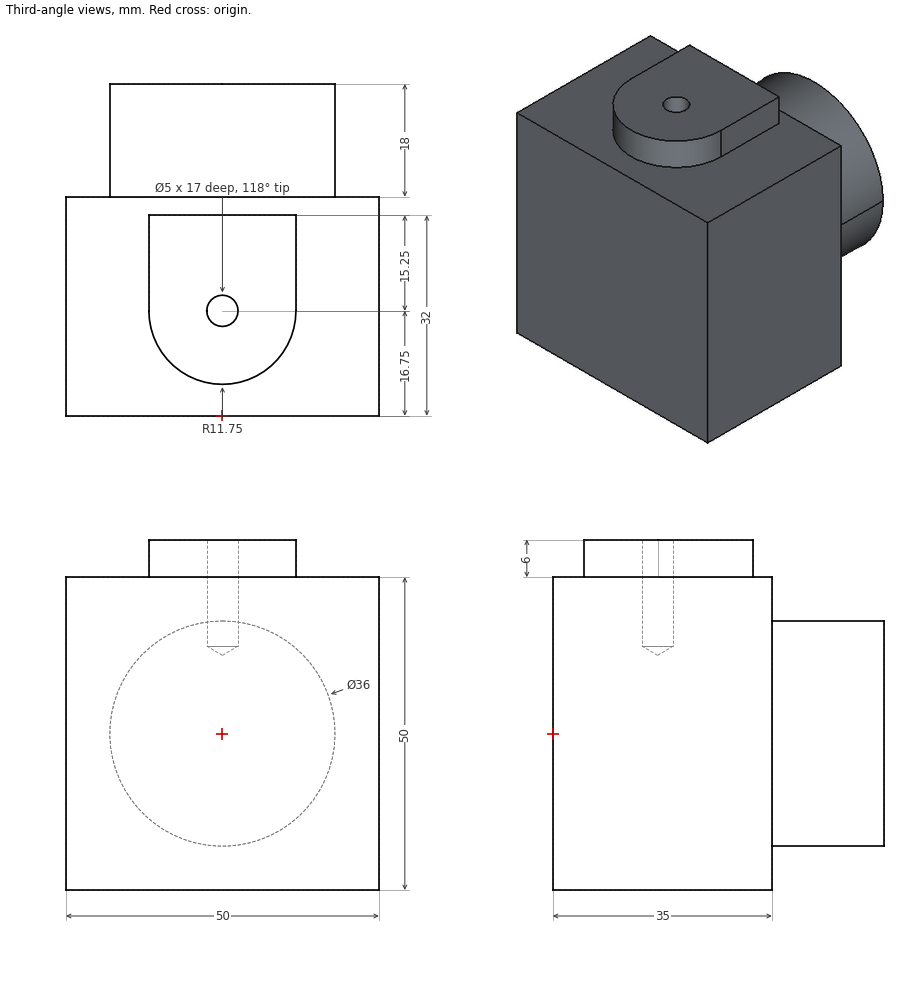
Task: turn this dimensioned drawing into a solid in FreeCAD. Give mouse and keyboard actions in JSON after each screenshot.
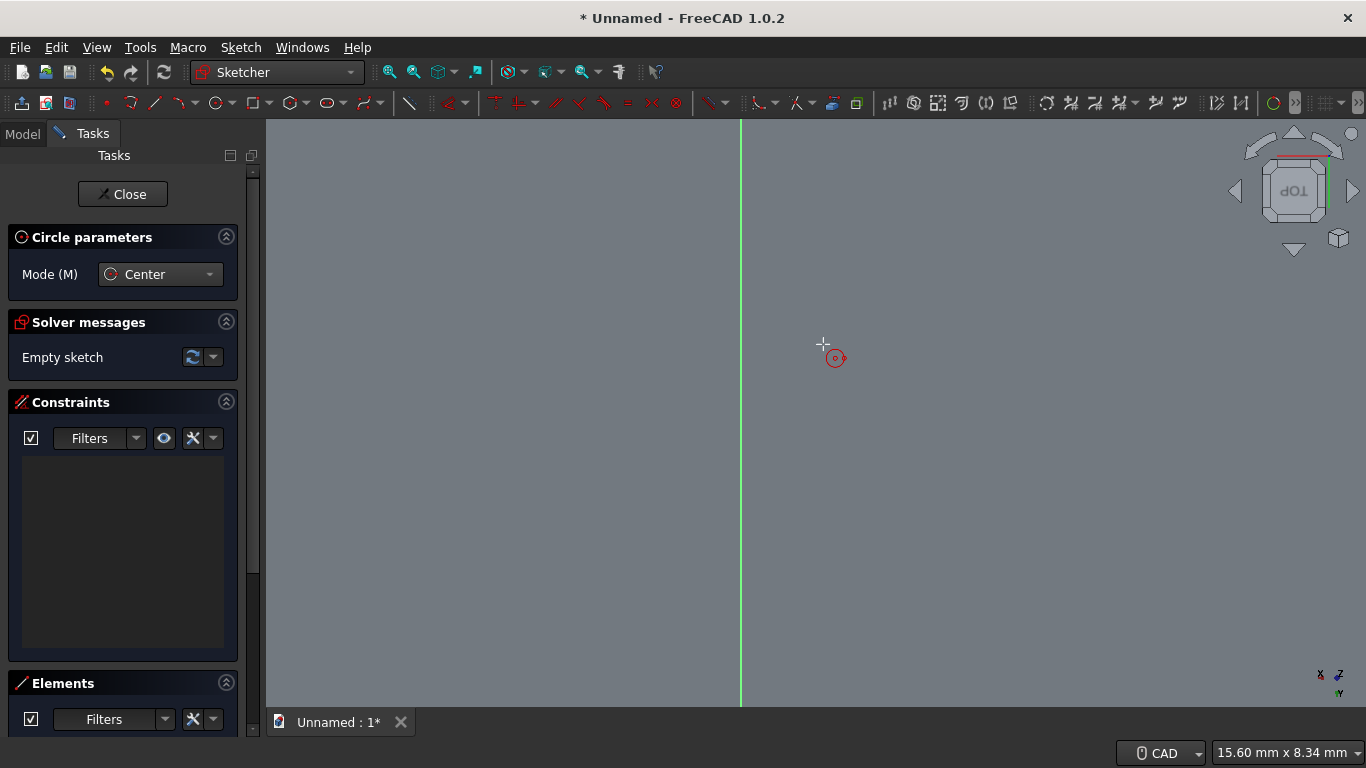
{"action": "left_click", "coordinate": [741, 413]}
{"action": "left_click", "coordinate": [865, 288]}
{"action": "key", "text": "Escape"}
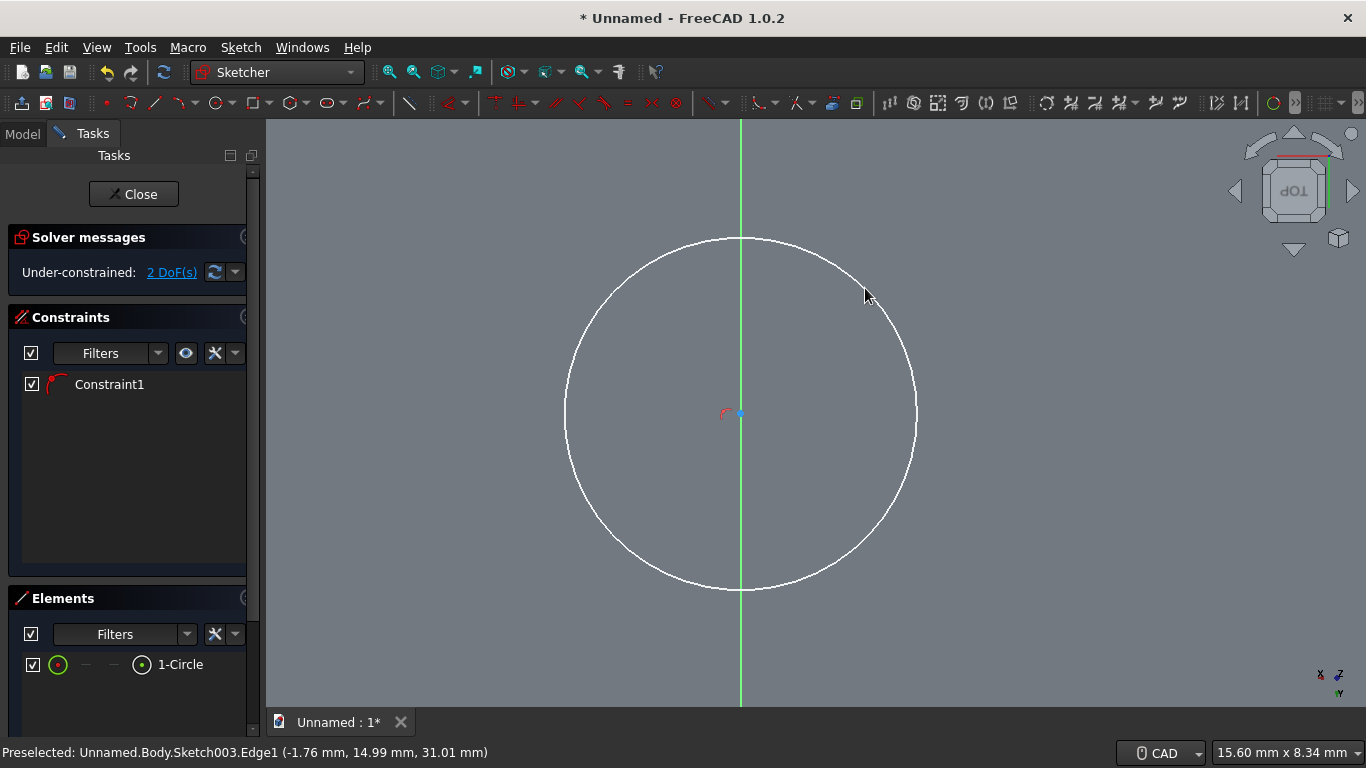
{"action": "key", "text": "d"}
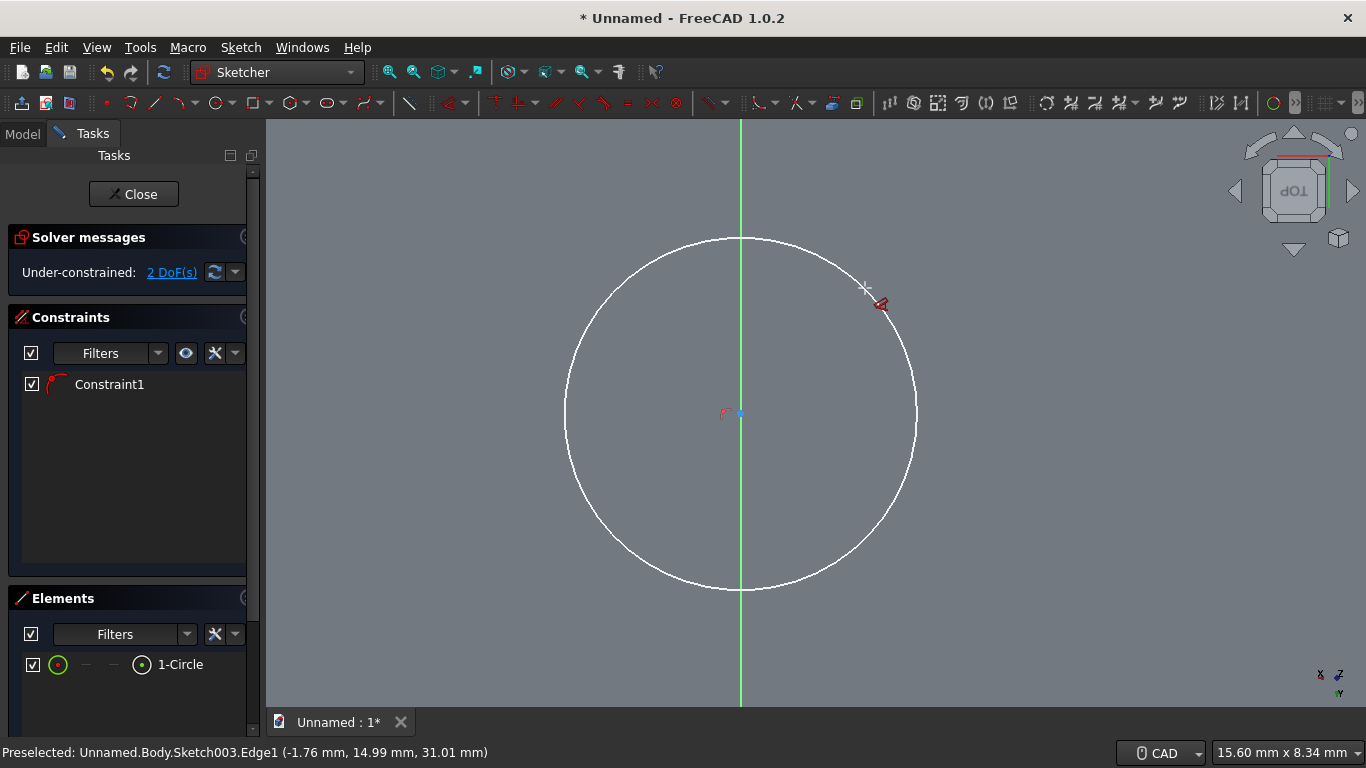
{"action": "left_click", "coordinate": [865, 289]}
{"action": "left_click", "coordinate": [888, 266]}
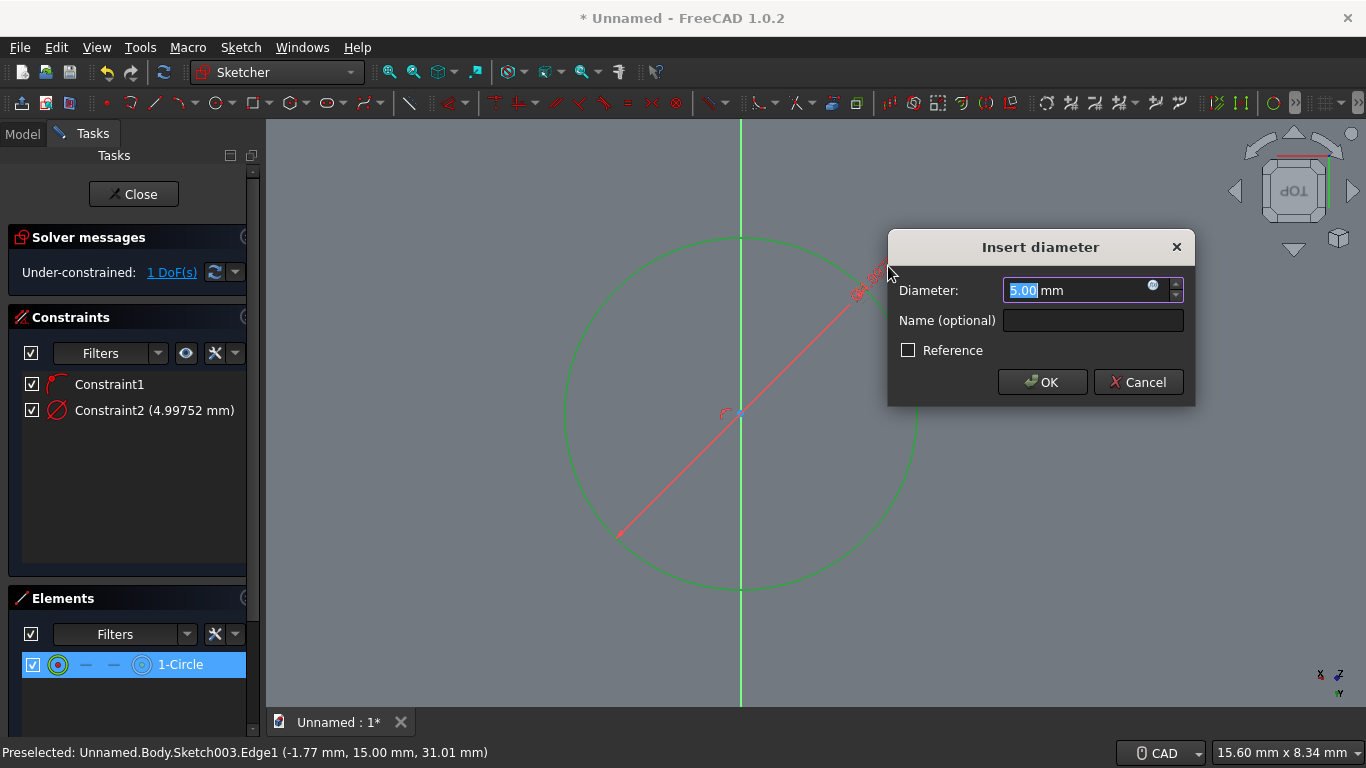
{"action": "type", "text": "5"}
{"action": "key", "text": "Return"}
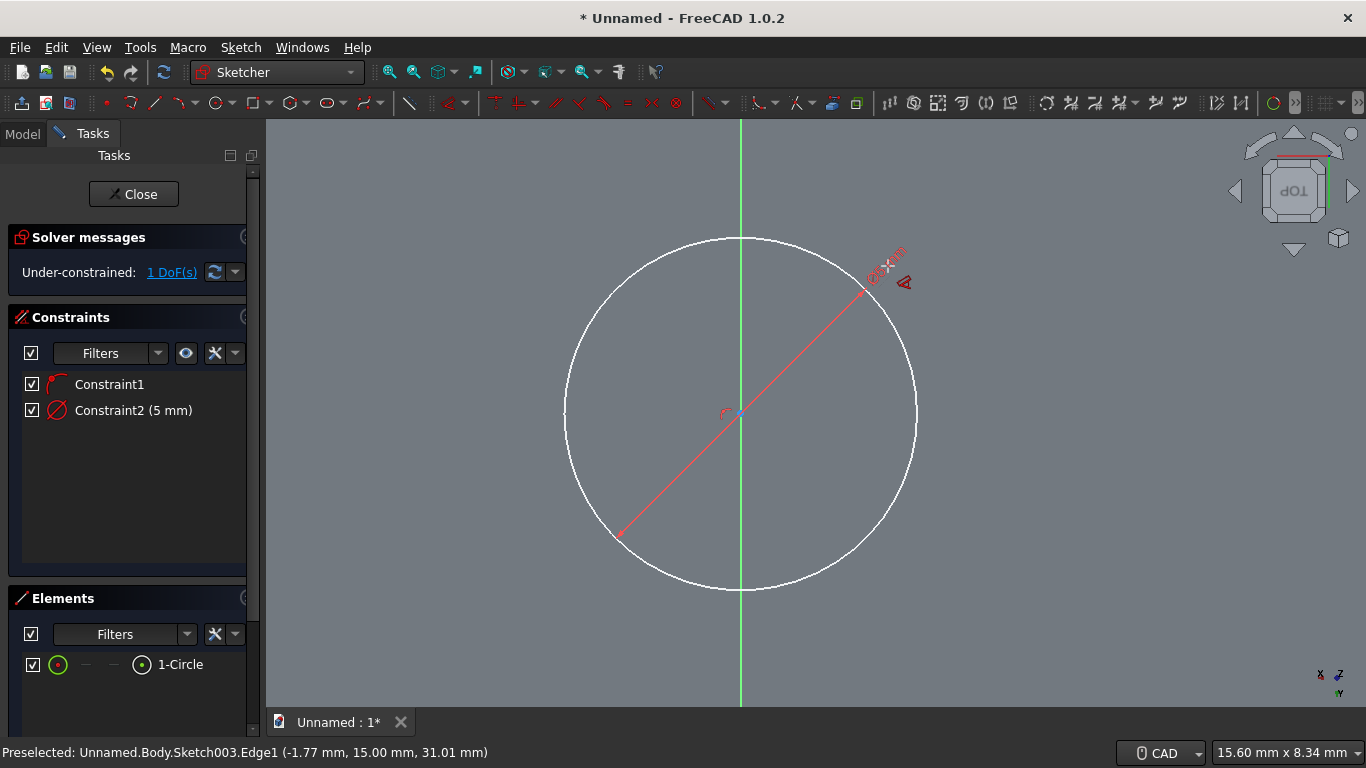
{"action": "left_click", "coordinate": [741, 414]}
{"action": "left_click", "coordinate": [775, 280]}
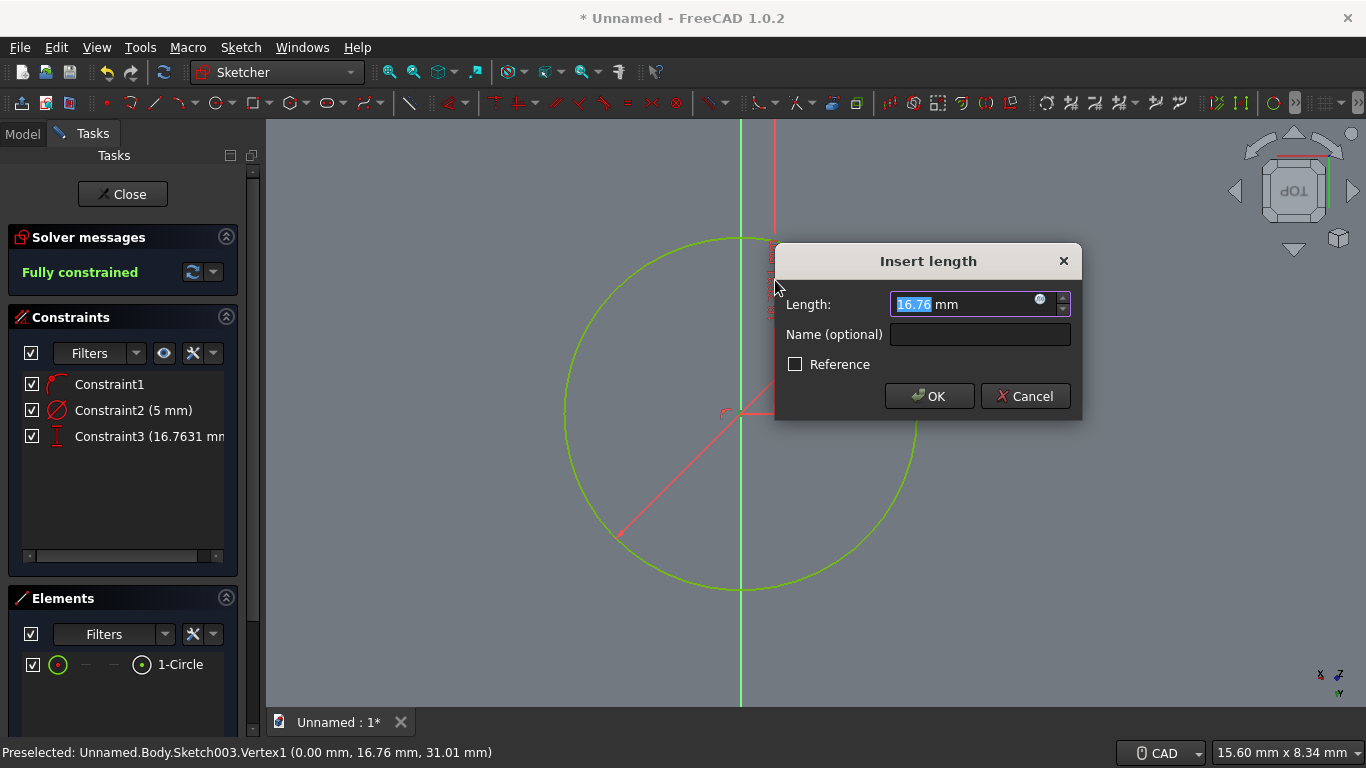
{"action": "type", "text": "16.75"}
{"action": "key", "text": "Return"}
{"action": "key", "text": "Escape"}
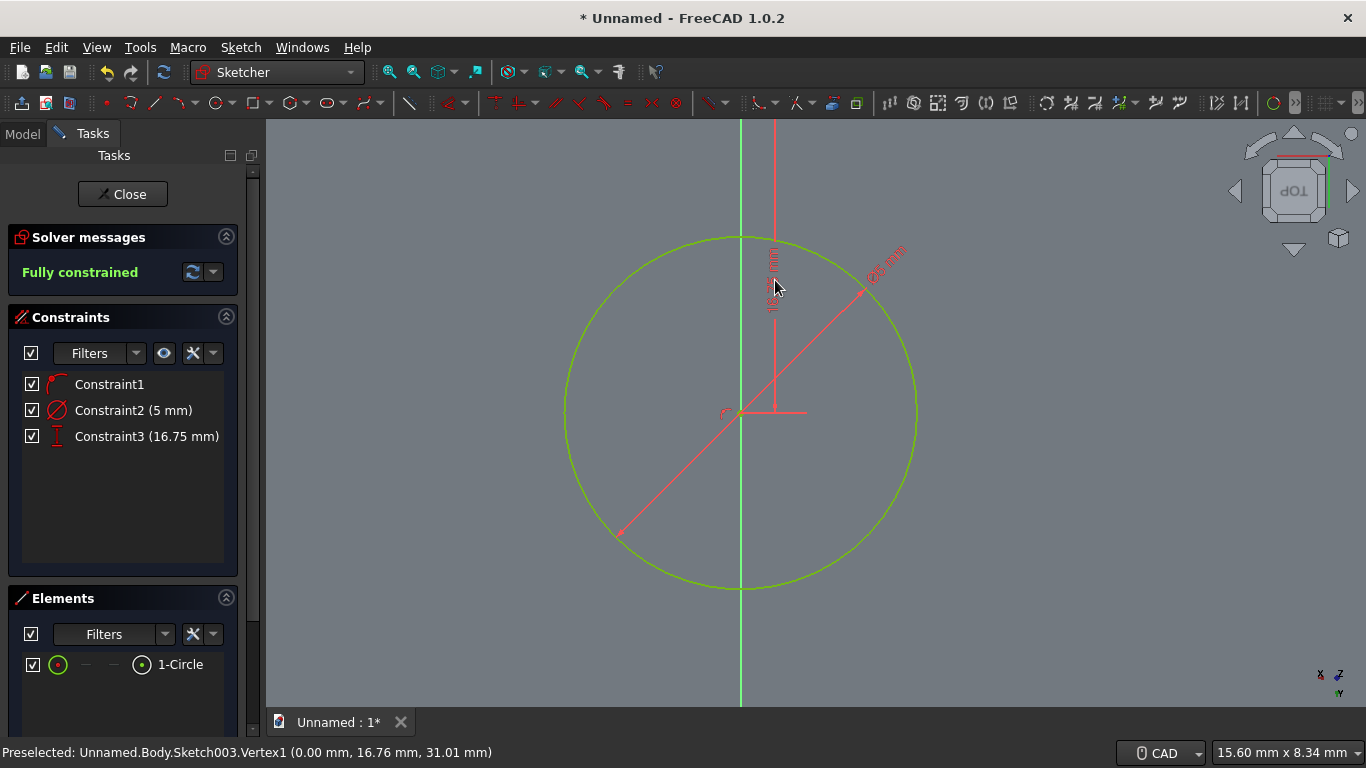
{"action": "left_click", "coordinate": [123, 194]}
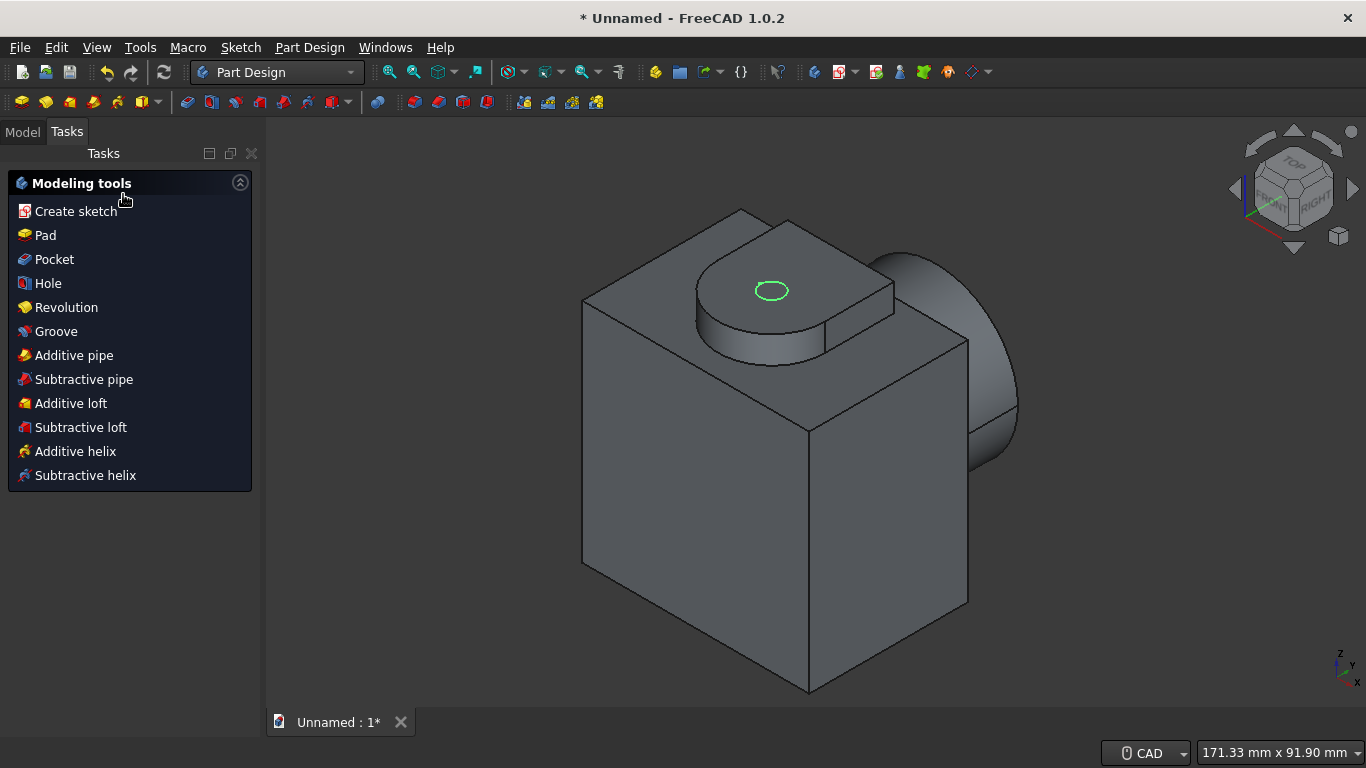
{"action": "left_click", "coordinate": [212, 102]}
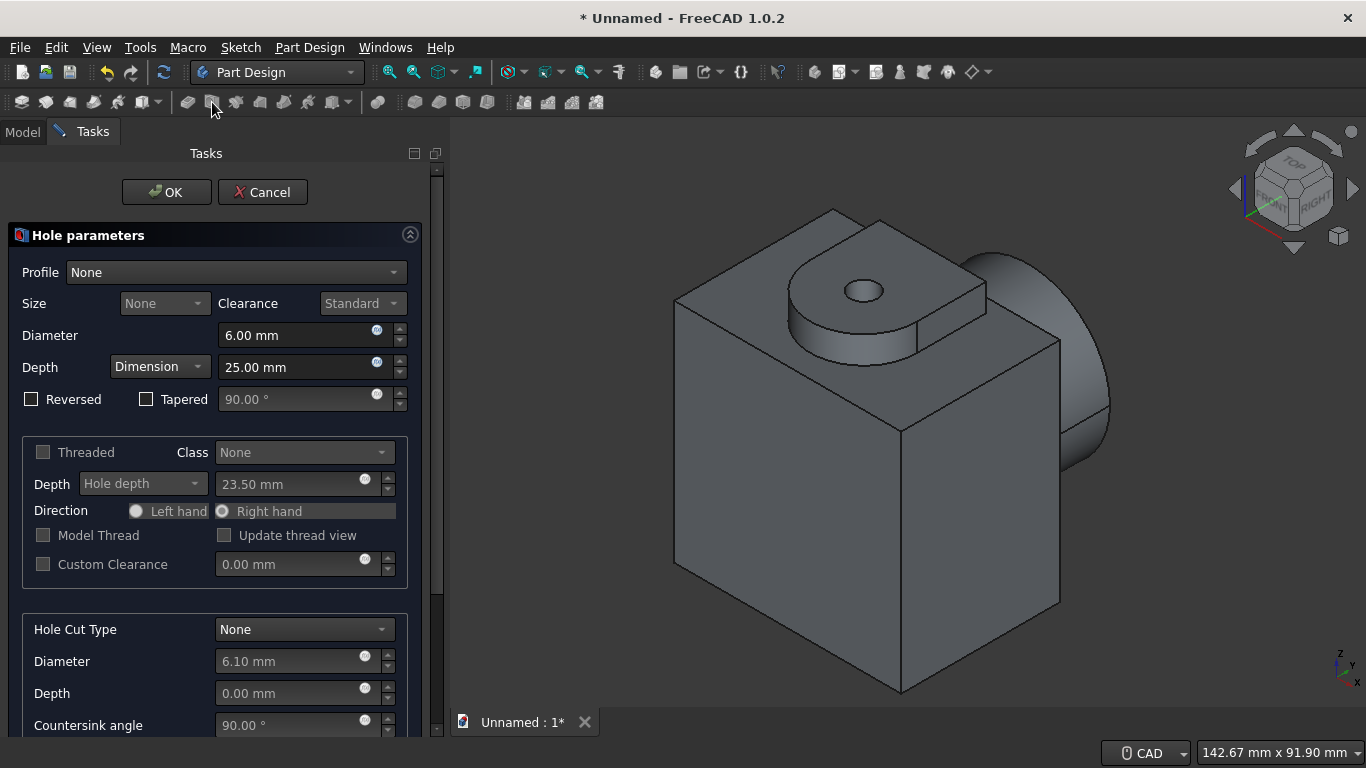
{"action": "triple_click", "coordinate": [305, 335]}